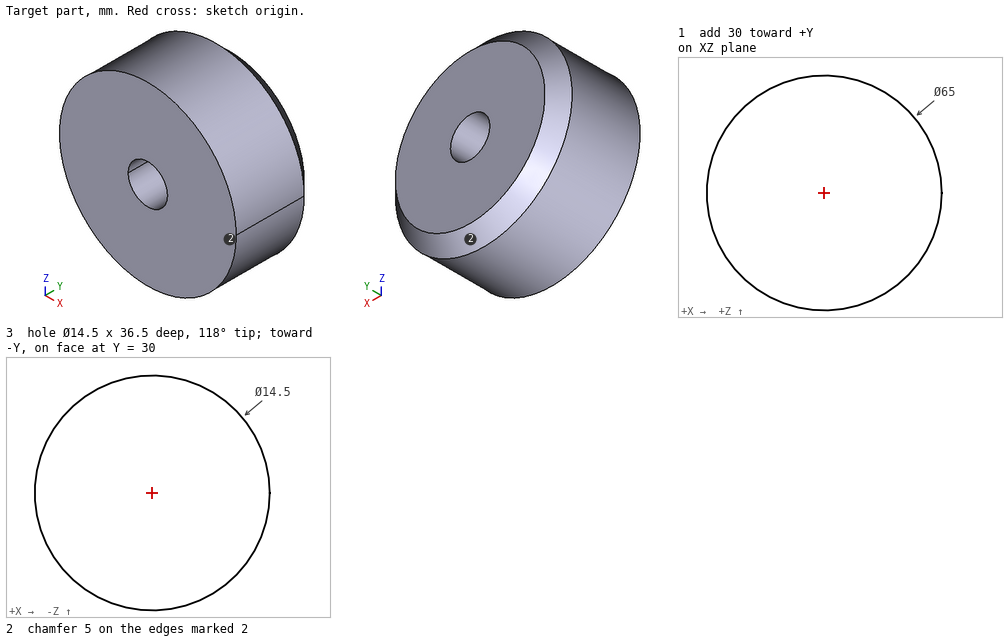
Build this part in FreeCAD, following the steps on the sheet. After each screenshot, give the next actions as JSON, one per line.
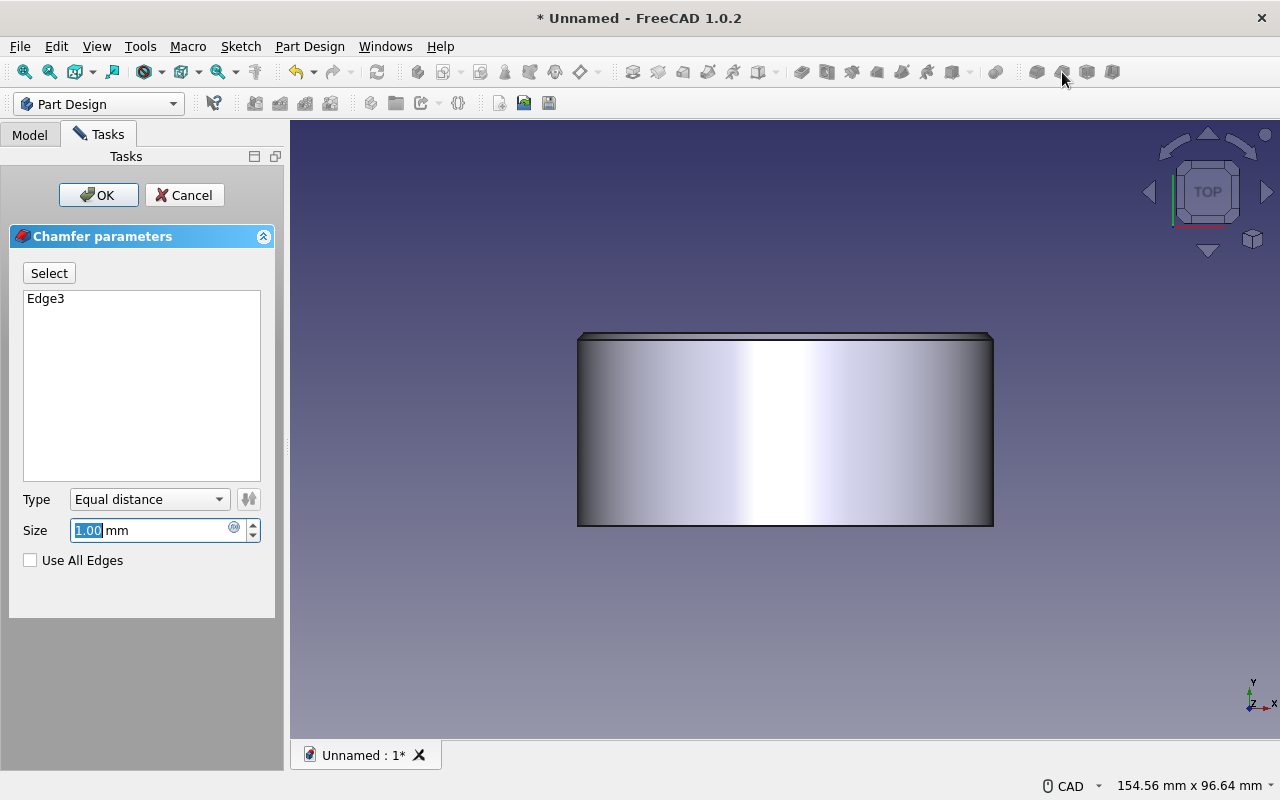
{"action": "type", "text": "5"}
{"action": "key", "text": "Tab"}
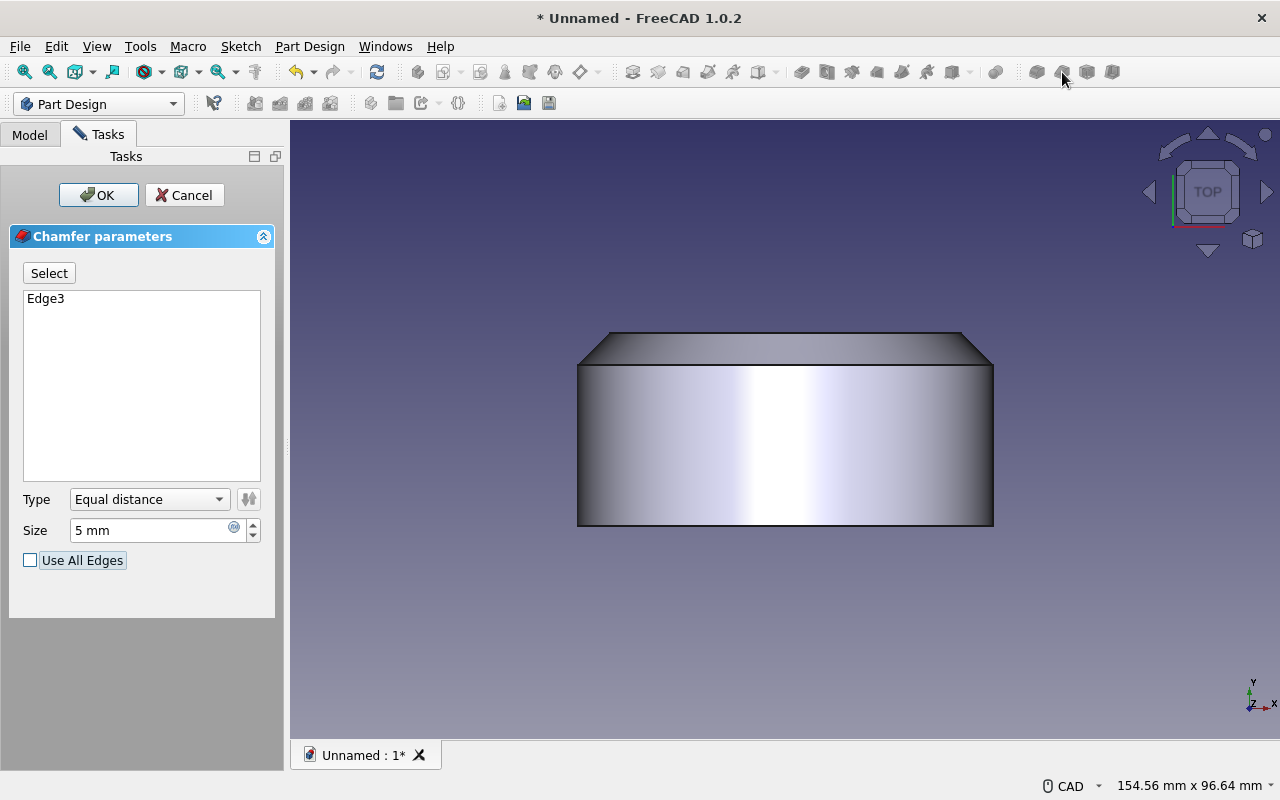
{"action": "left_click", "coordinate": [99, 195]}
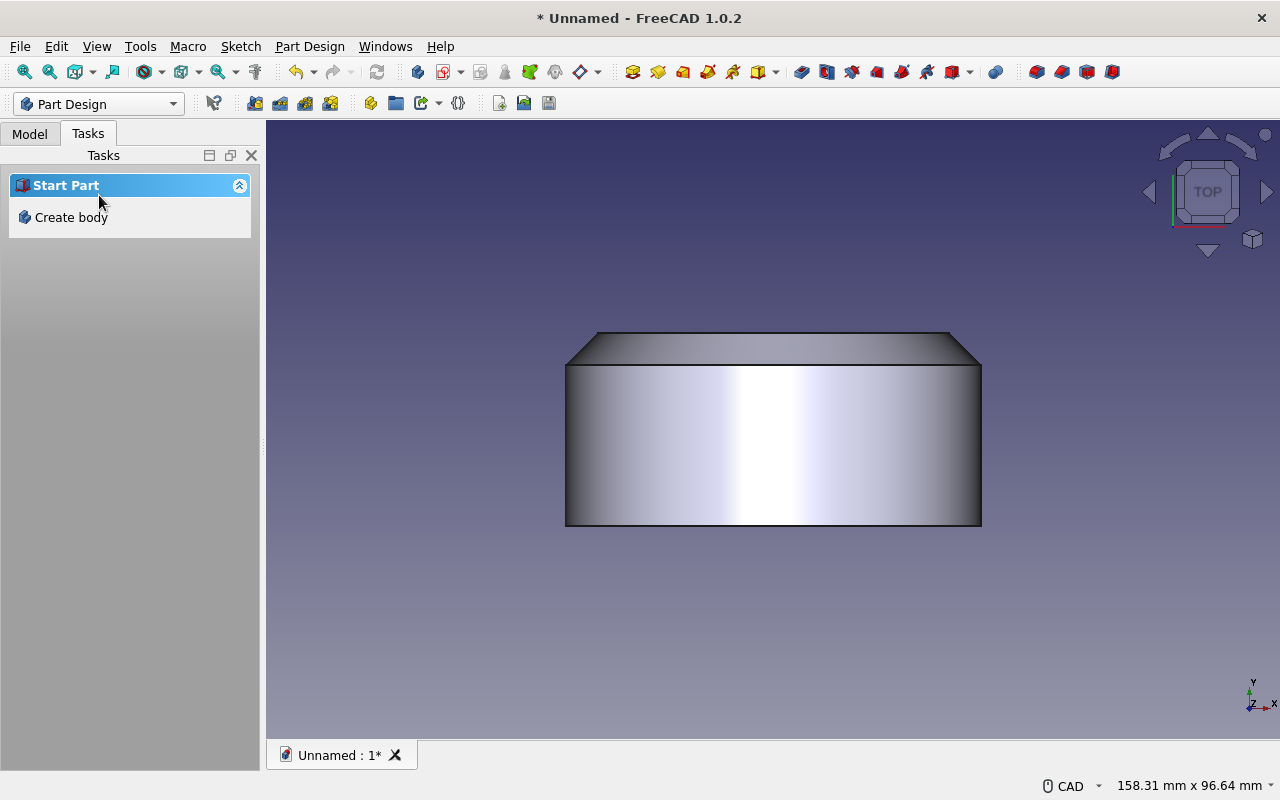
{"action": "left_click", "coordinate": [25, 72]}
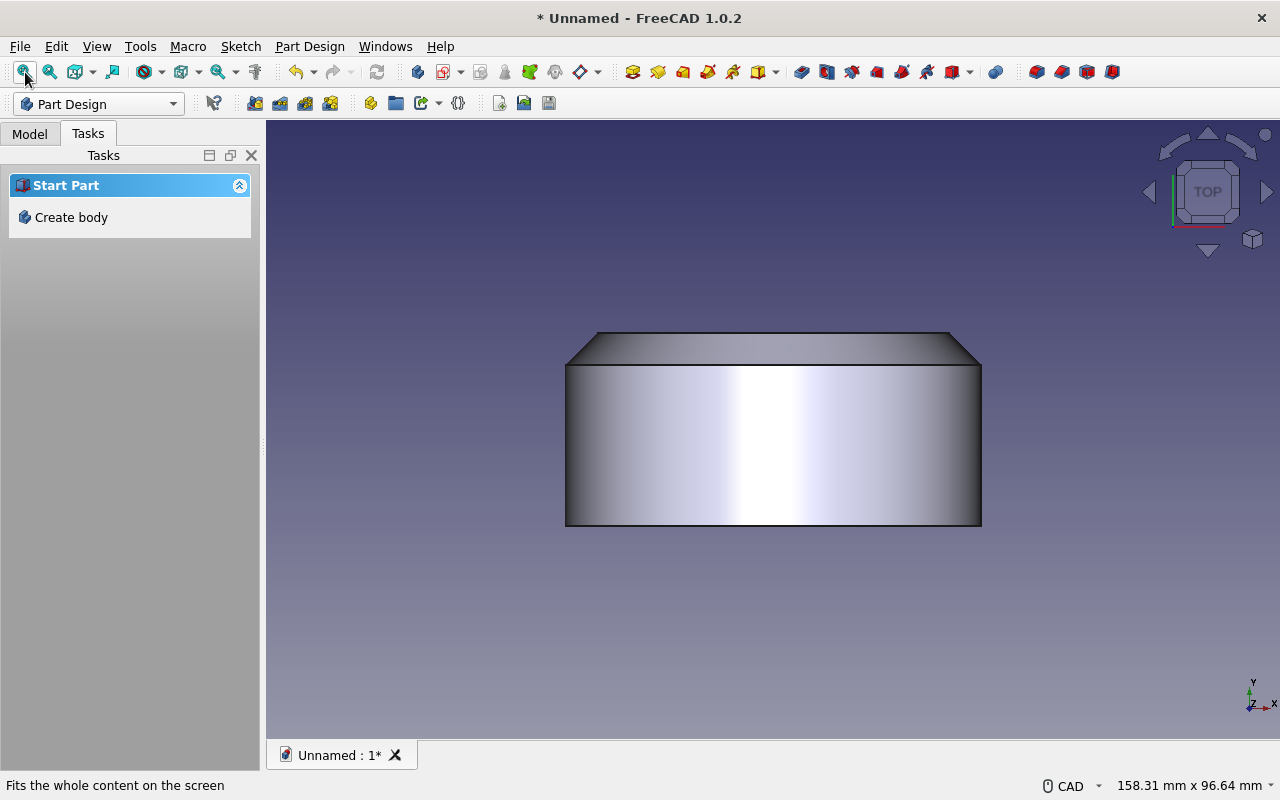
{"action": "key", "text": "4"}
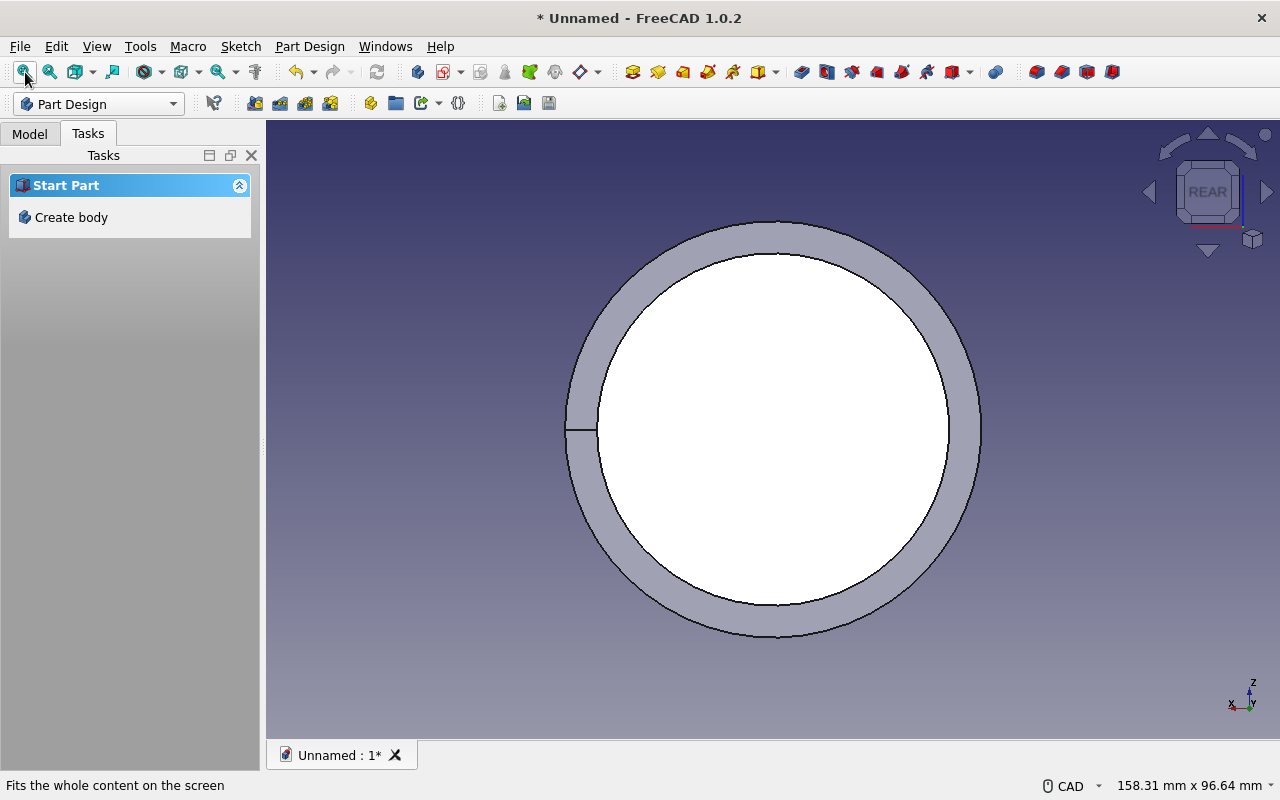
{"action": "left_click", "coordinate": [773, 428]}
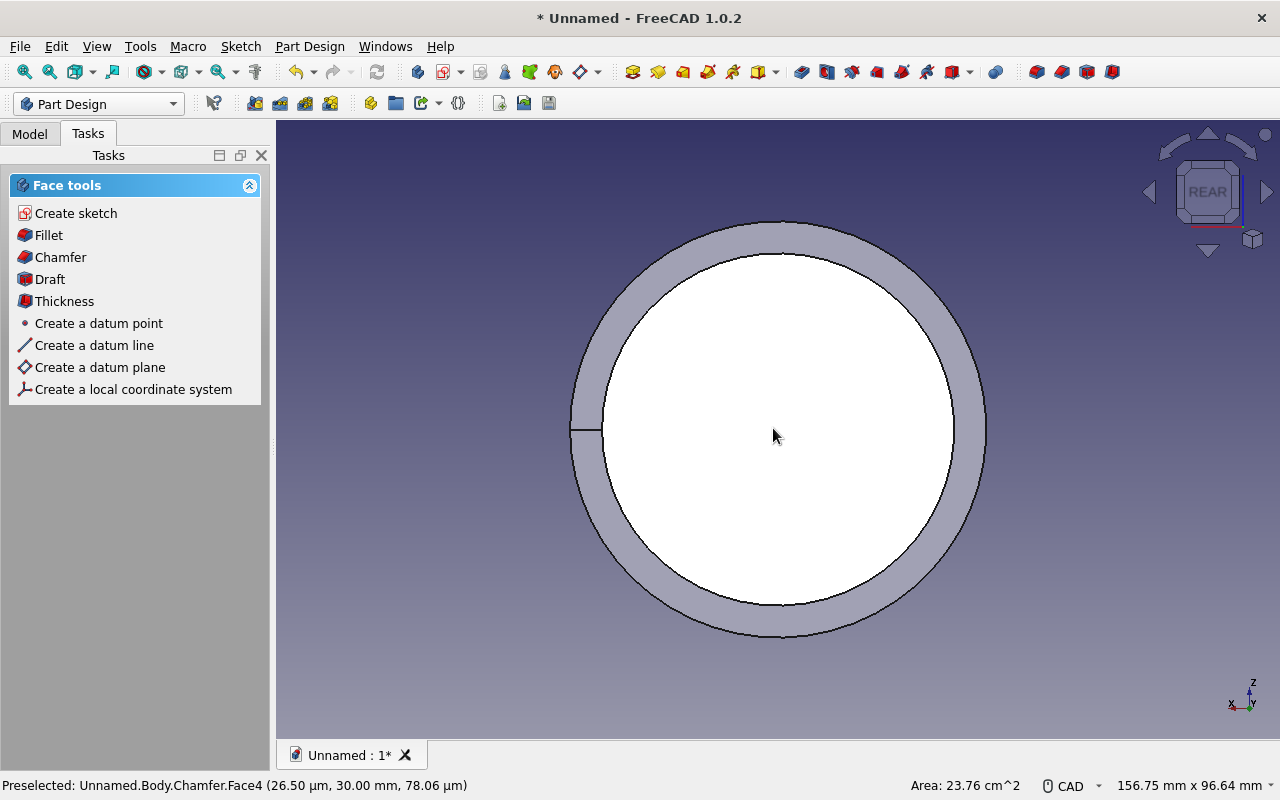
{"action": "left_click", "coordinate": [442, 72]}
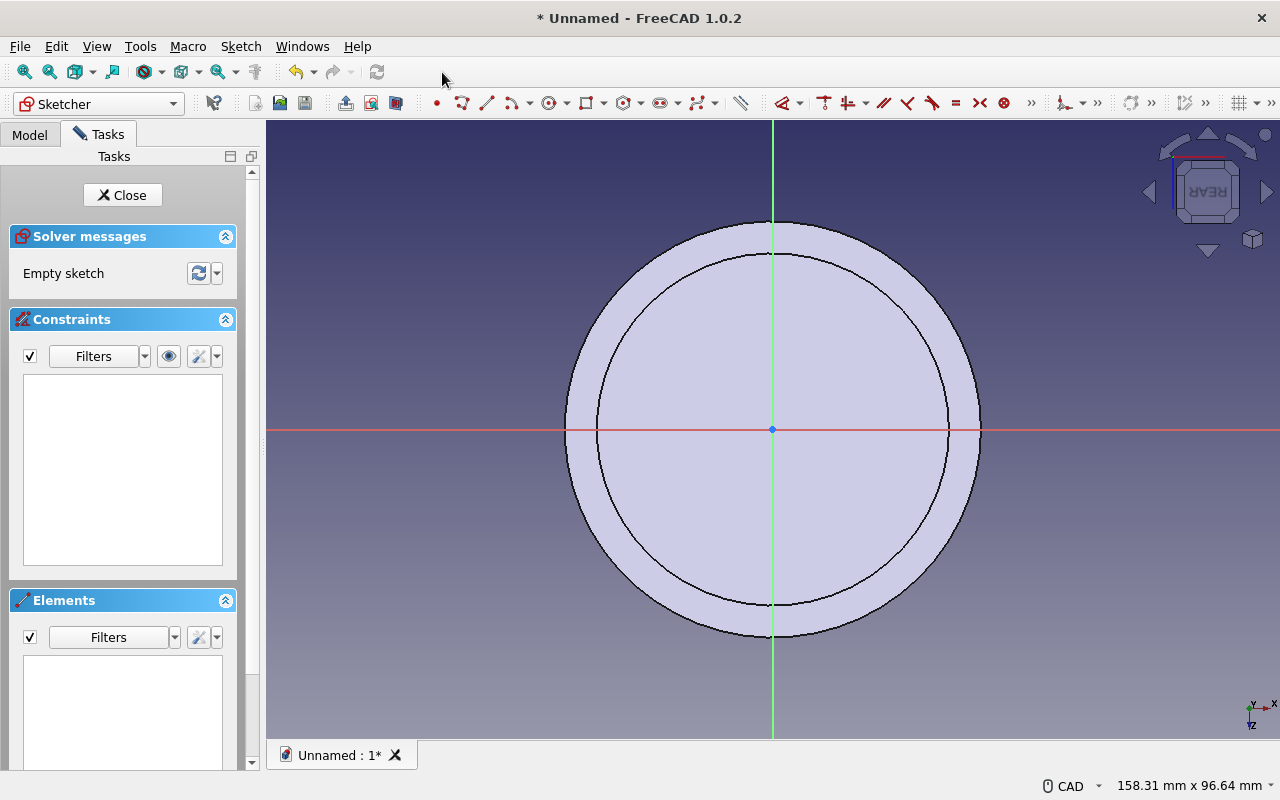
{"action": "scroll", "coordinate": [795, 430], "scroll_direction": "up", "scroll_amount": 7}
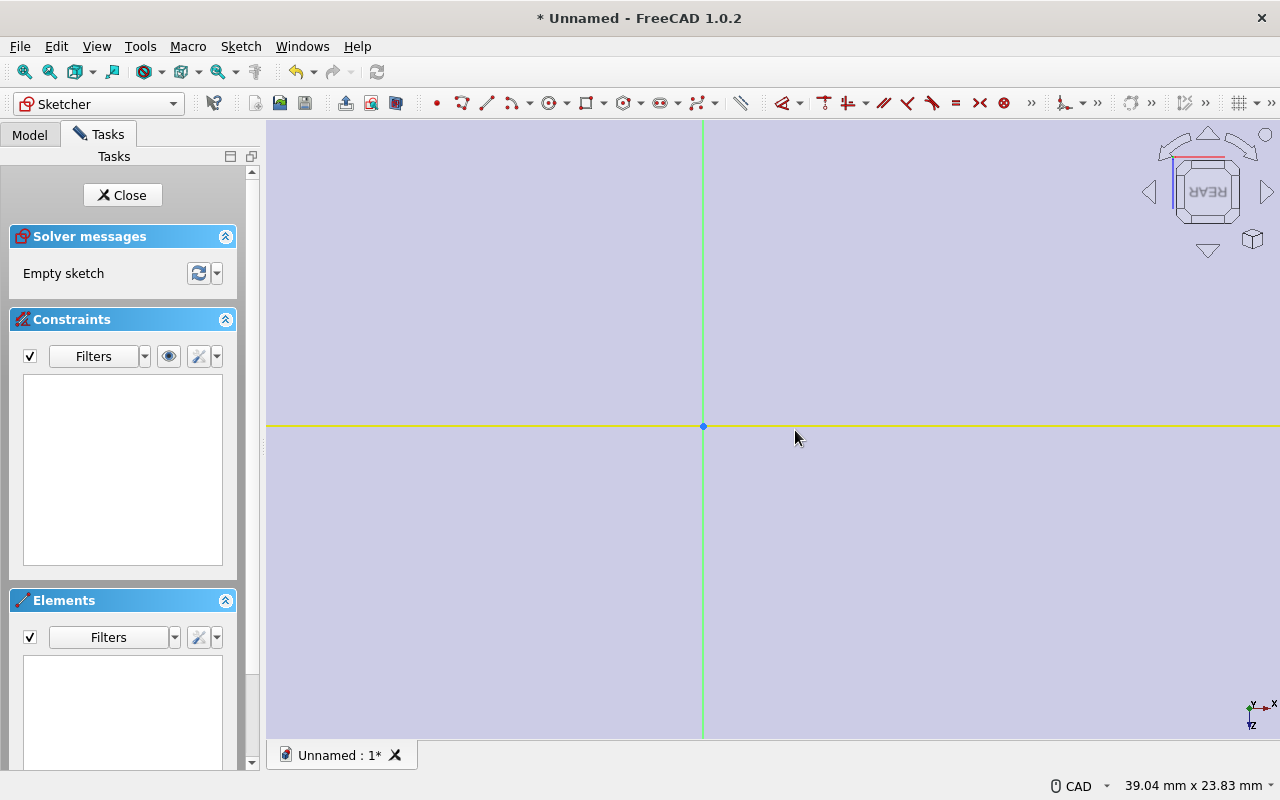
{"action": "left_click", "coordinate": [548, 104]}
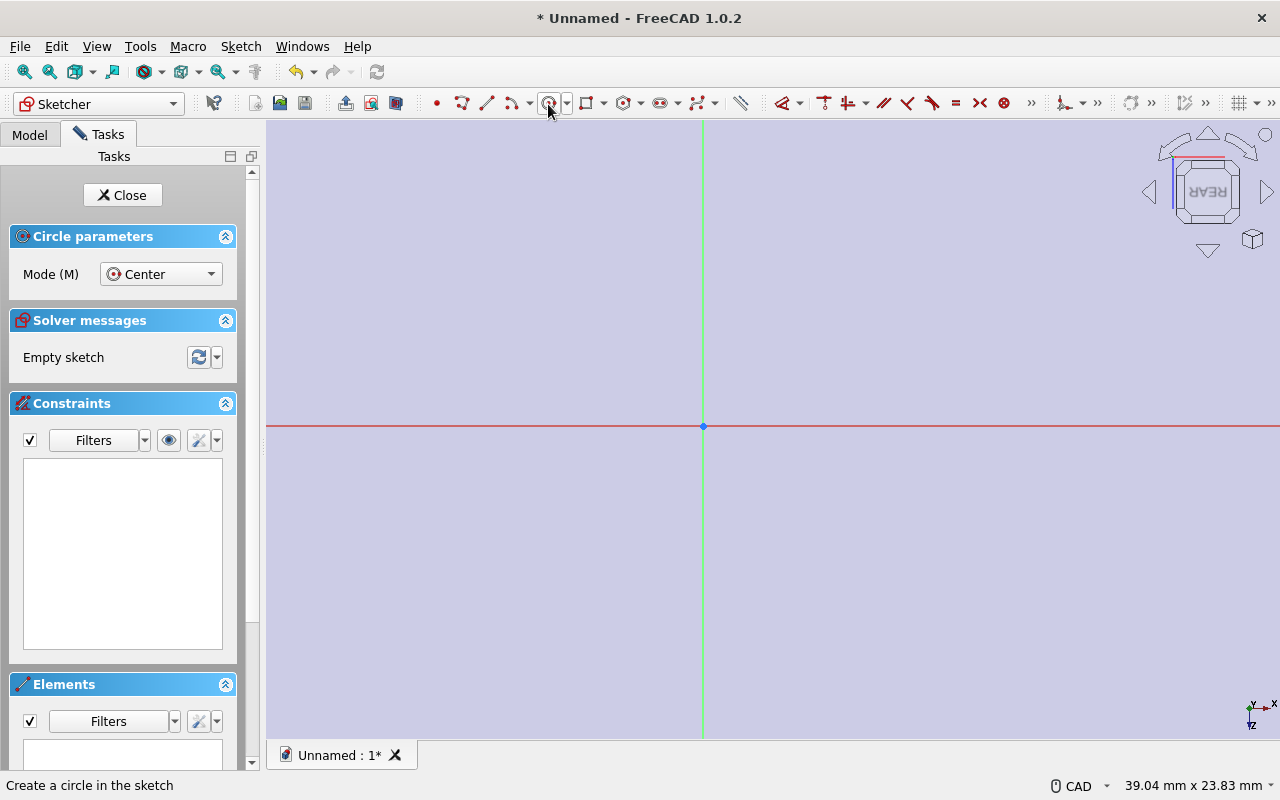
{"action": "left_click", "coordinate": [704, 426]}
{"action": "left_click", "coordinate": [837, 293]}
{"action": "key", "text": "Escape"}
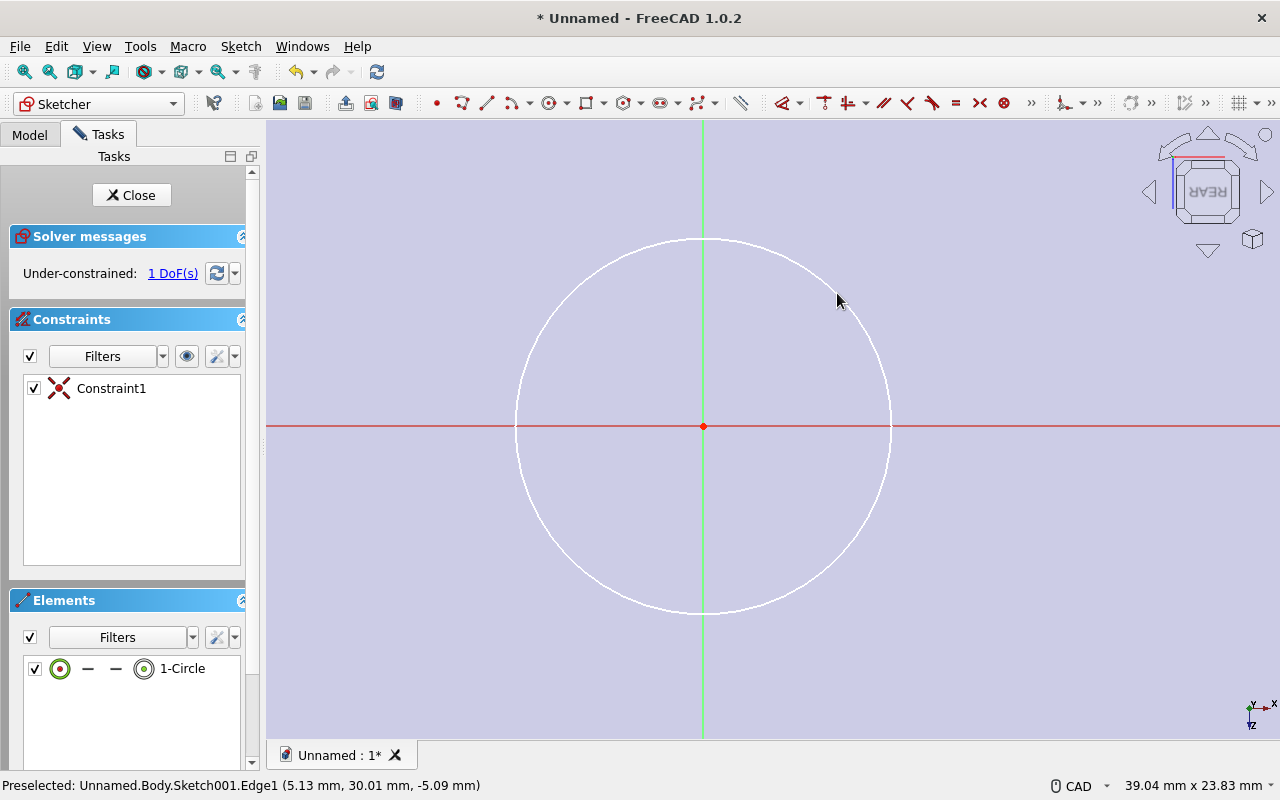
{"action": "left_click", "coordinate": [782, 104]}